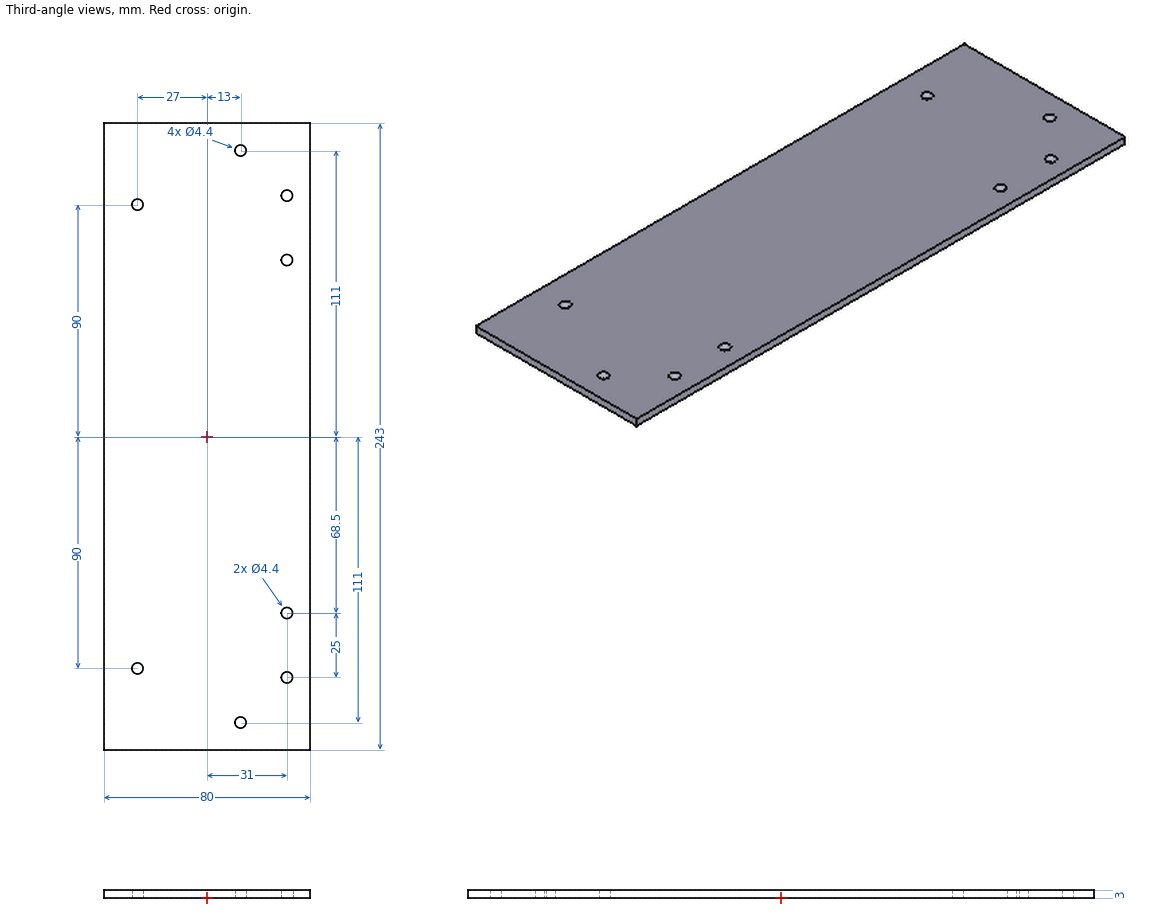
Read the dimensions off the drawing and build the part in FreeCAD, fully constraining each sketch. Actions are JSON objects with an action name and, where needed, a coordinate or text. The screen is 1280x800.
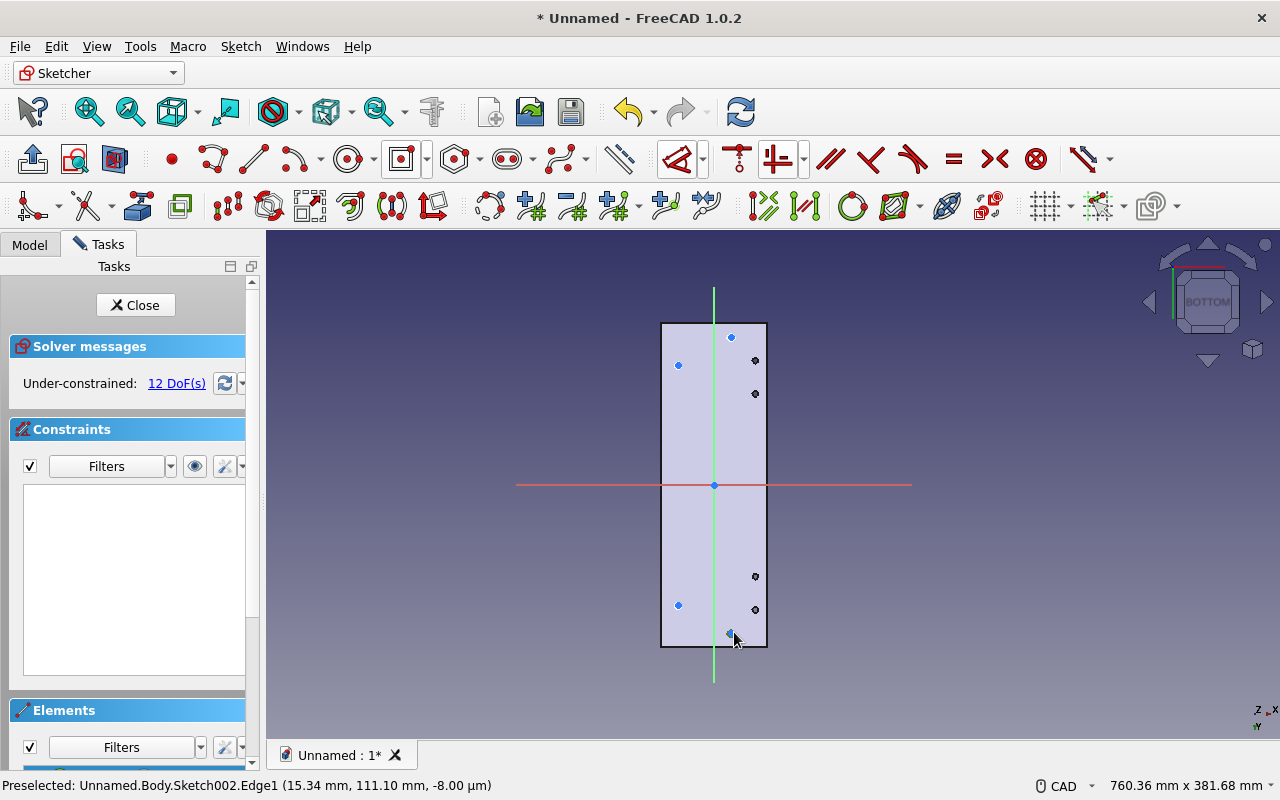
{"action": "scroll", "coordinate": [734, 335], "scroll_direction": "up", "scroll_amount": 7}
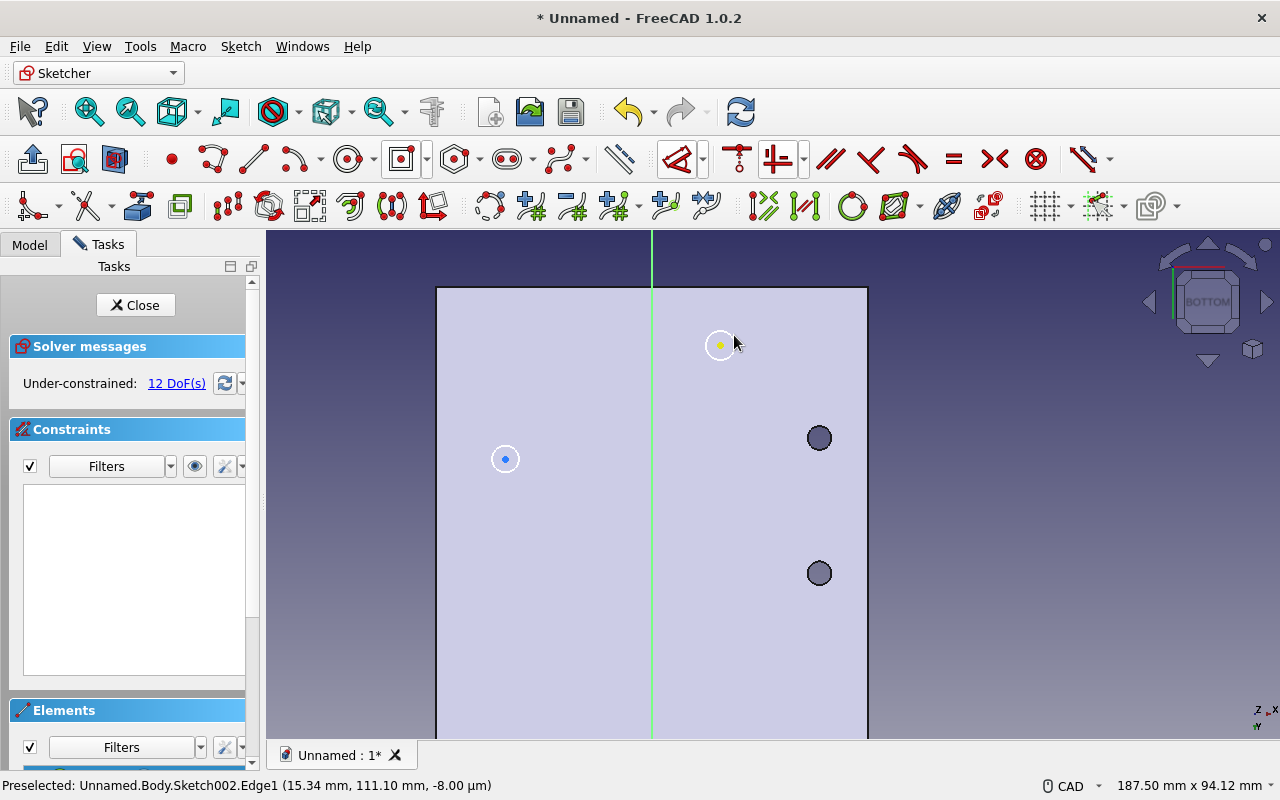
{"action": "left_click", "coordinate": [731, 335]}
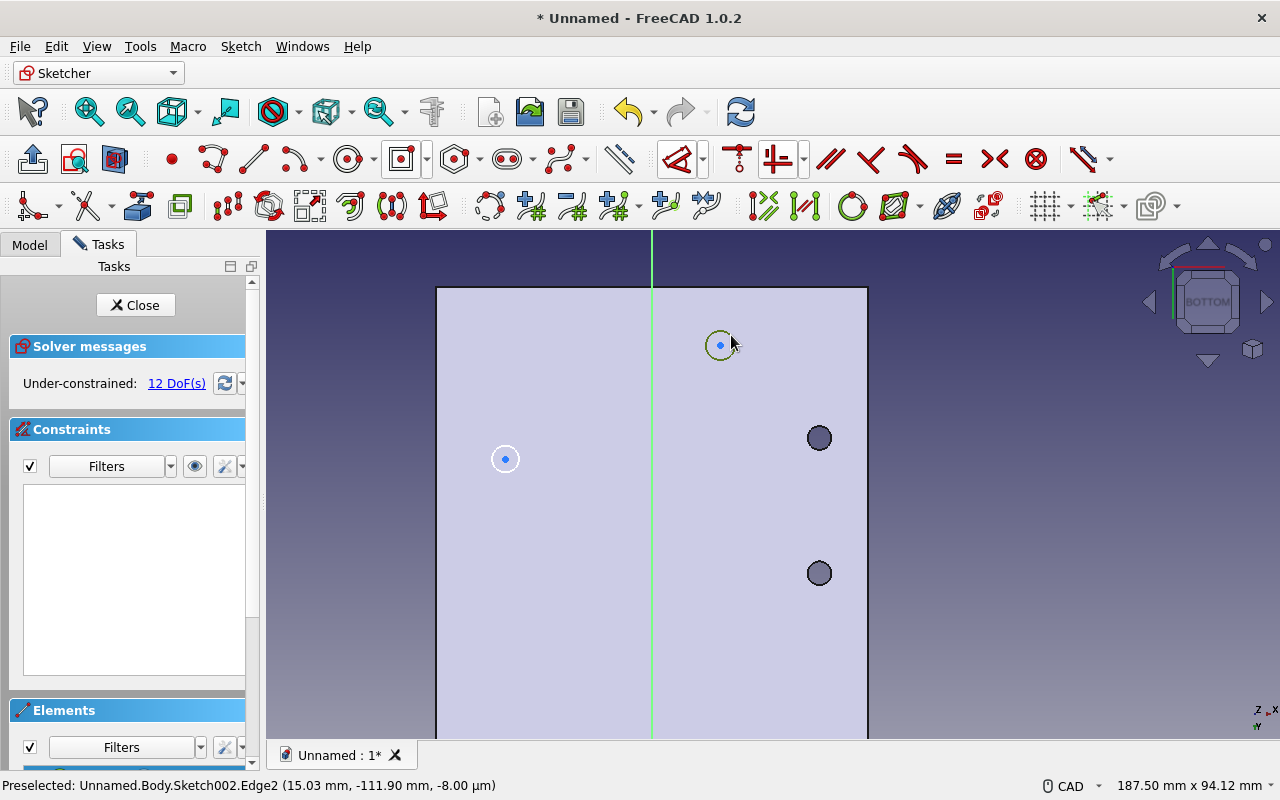
{"action": "scroll", "coordinate": [734, 334], "scroll_direction": "down", "scroll_amount": 7}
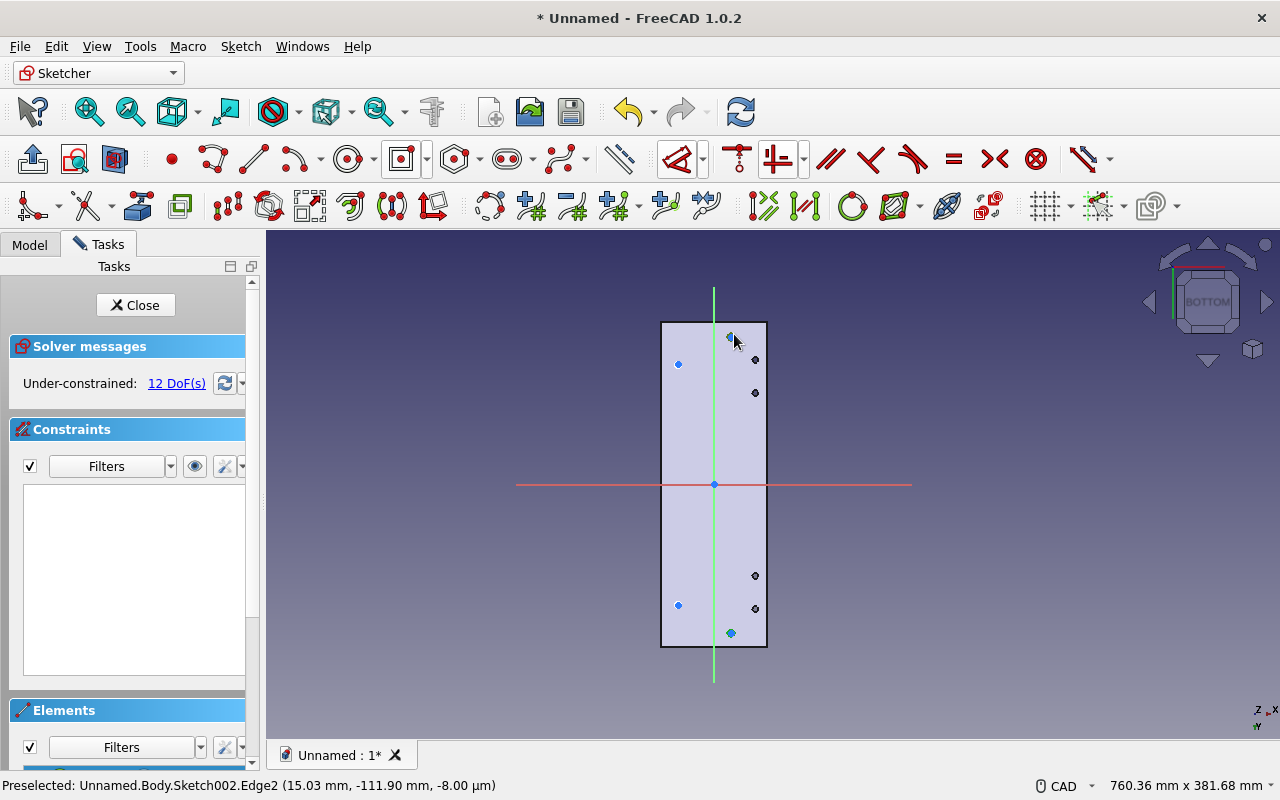
{"action": "scroll", "coordinate": [680, 603], "scroll_direction": "up", "scroll_amount": 8}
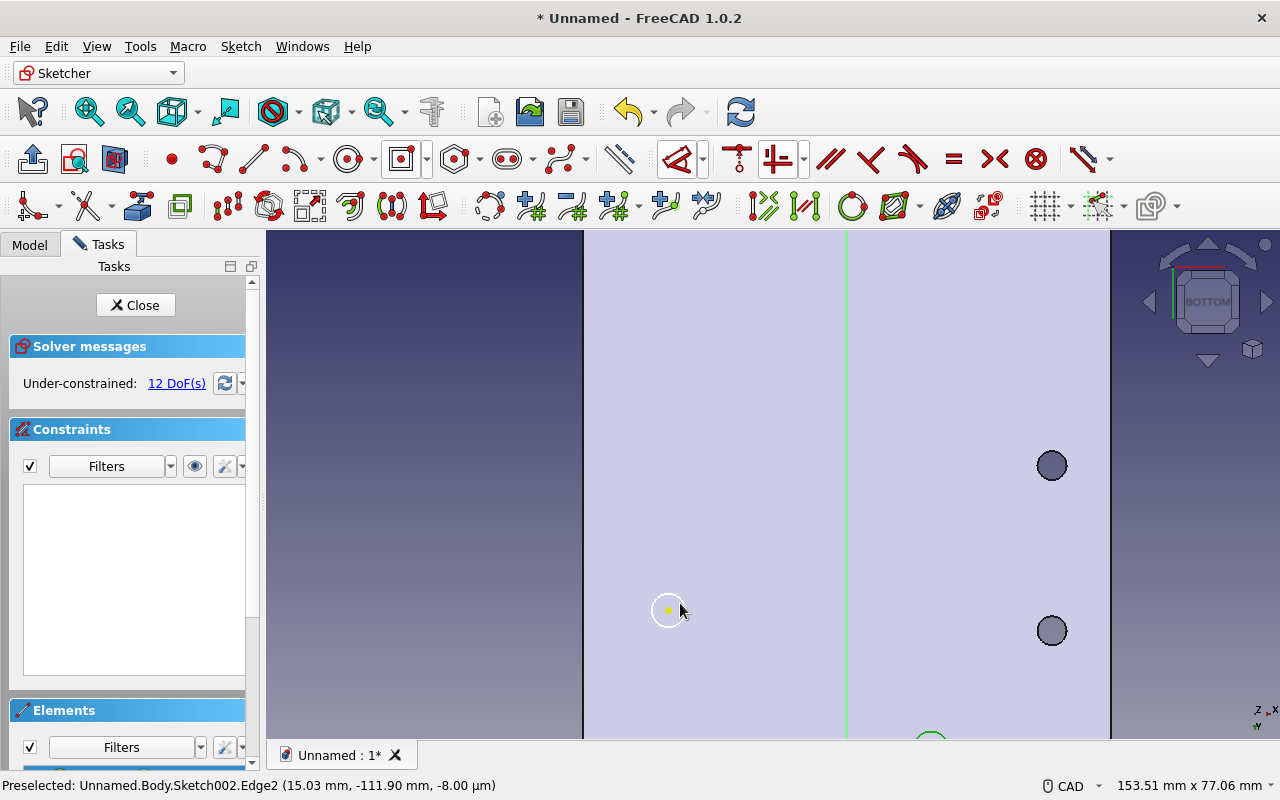
{"action": "left_click", "coordinate": [680, 599]}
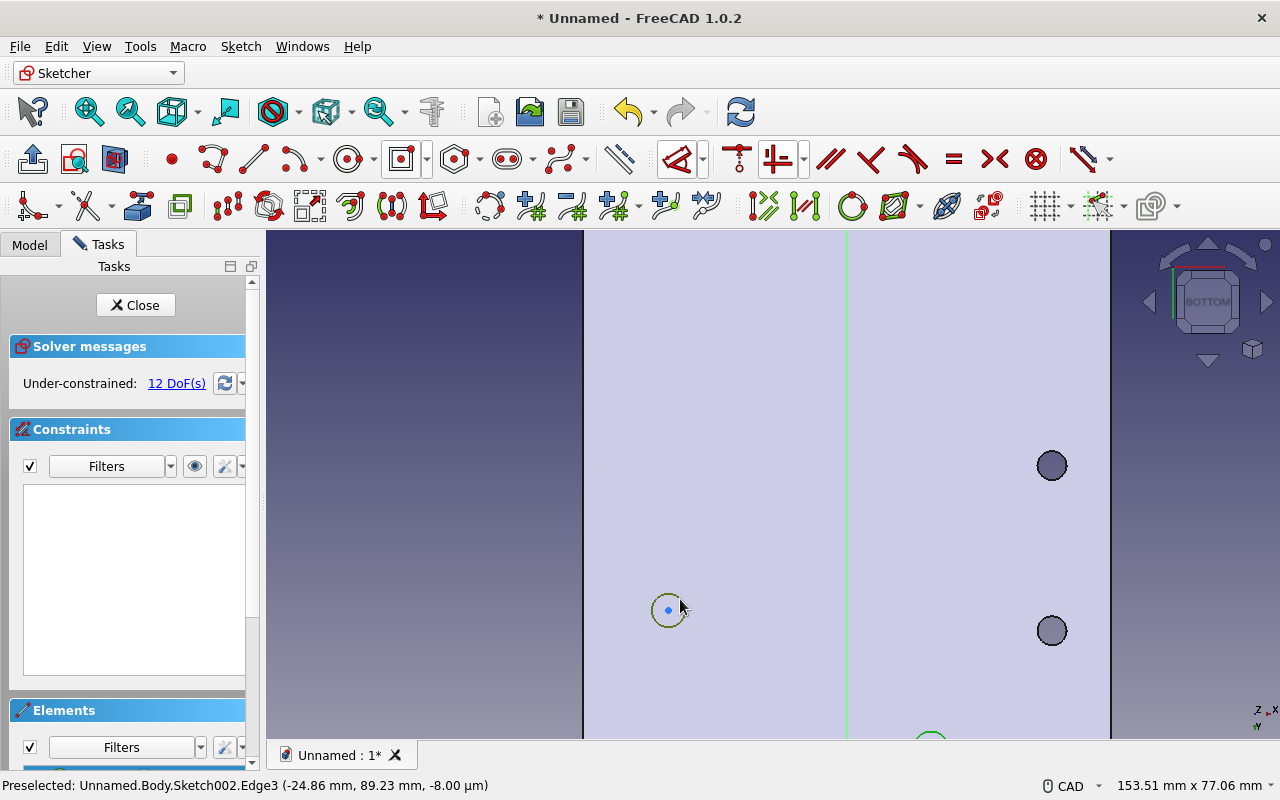
{"action": "scroll", "coordinate": [680, 604], "scroll_direction": "down", "scroll_amount": 8}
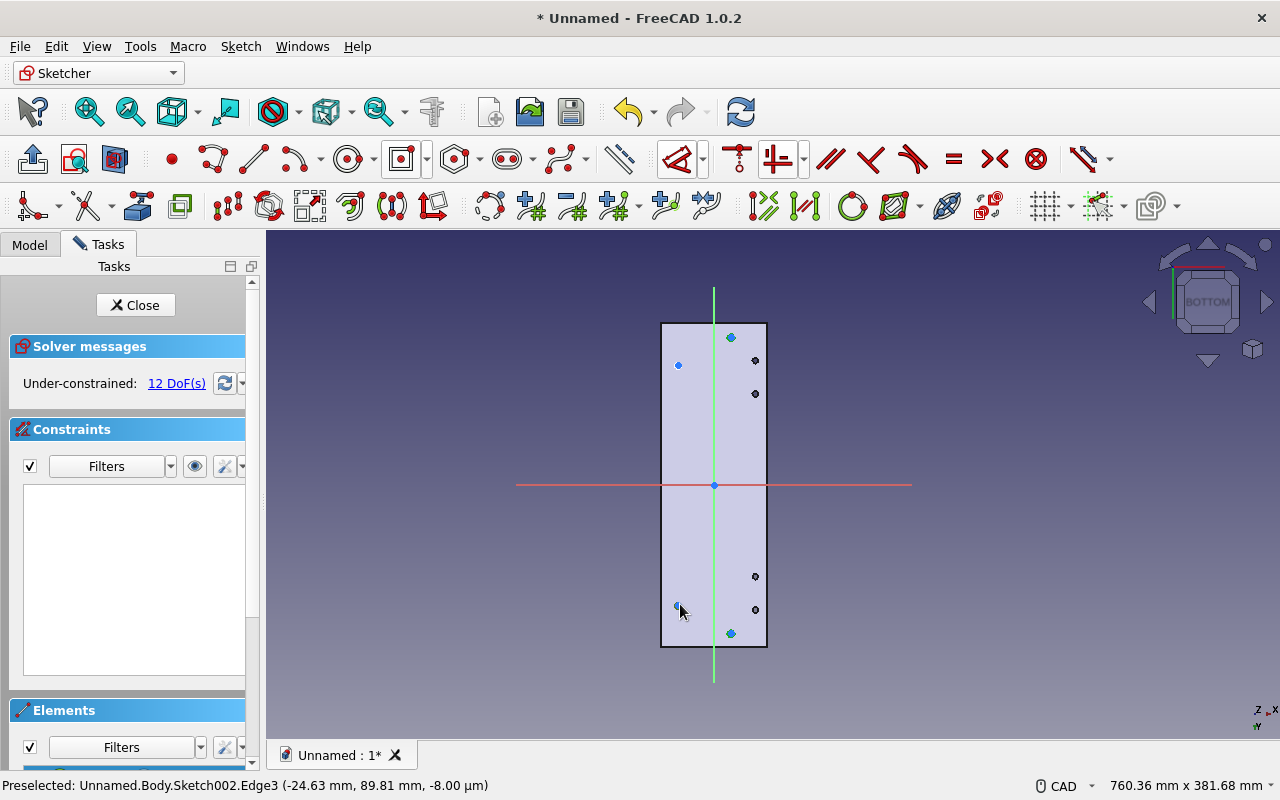
{"action": "scroll", "coordinate": [680, 363], "scroll_direction": "up", "scroll_amount": 8}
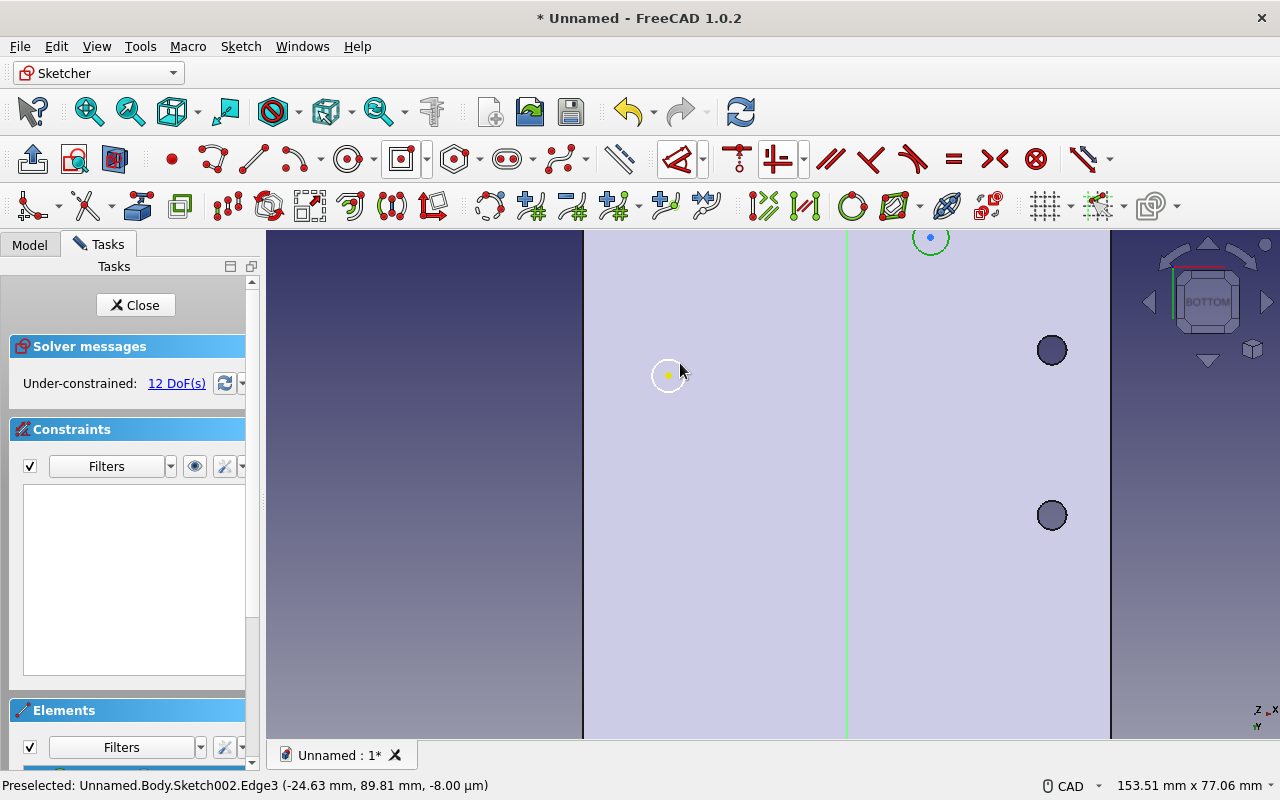
{"action": "left_click", "coordinate": [680, 364]}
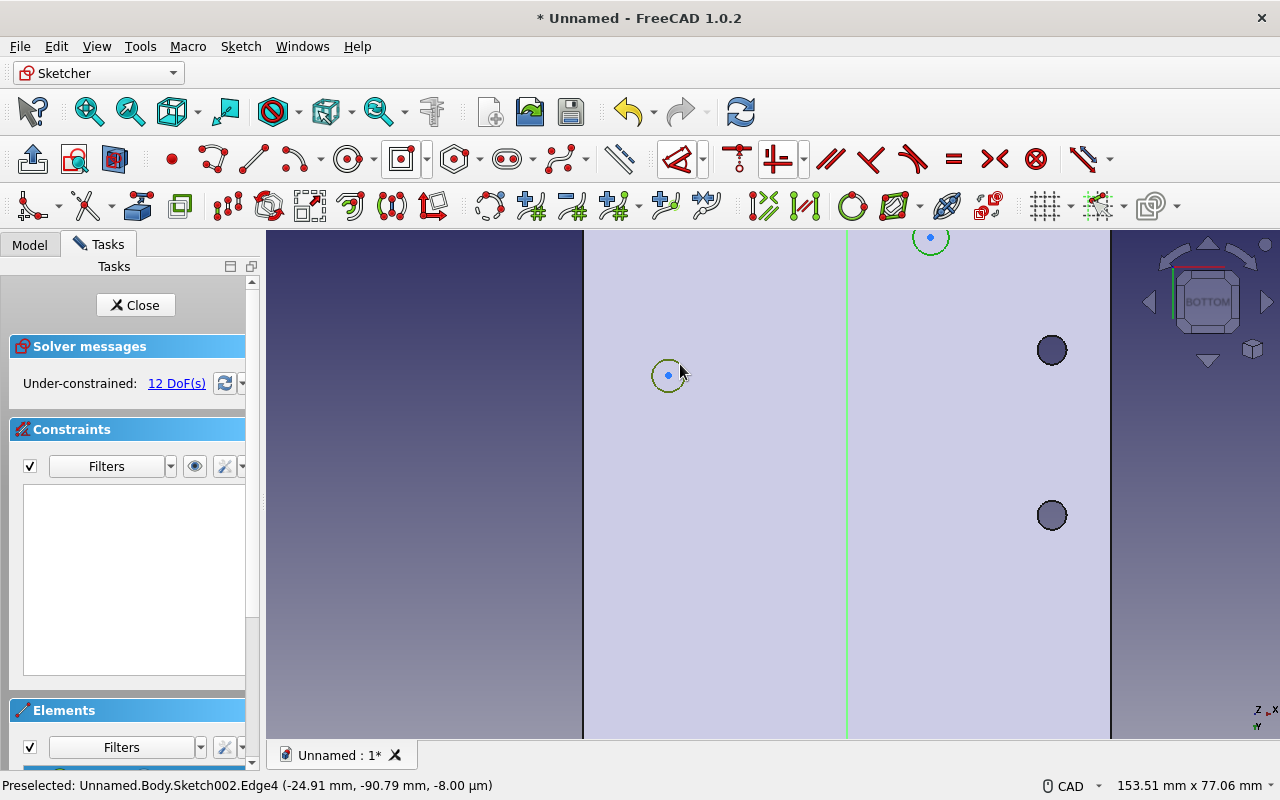
{"action": "left_click", "coordinate": [954, 160]}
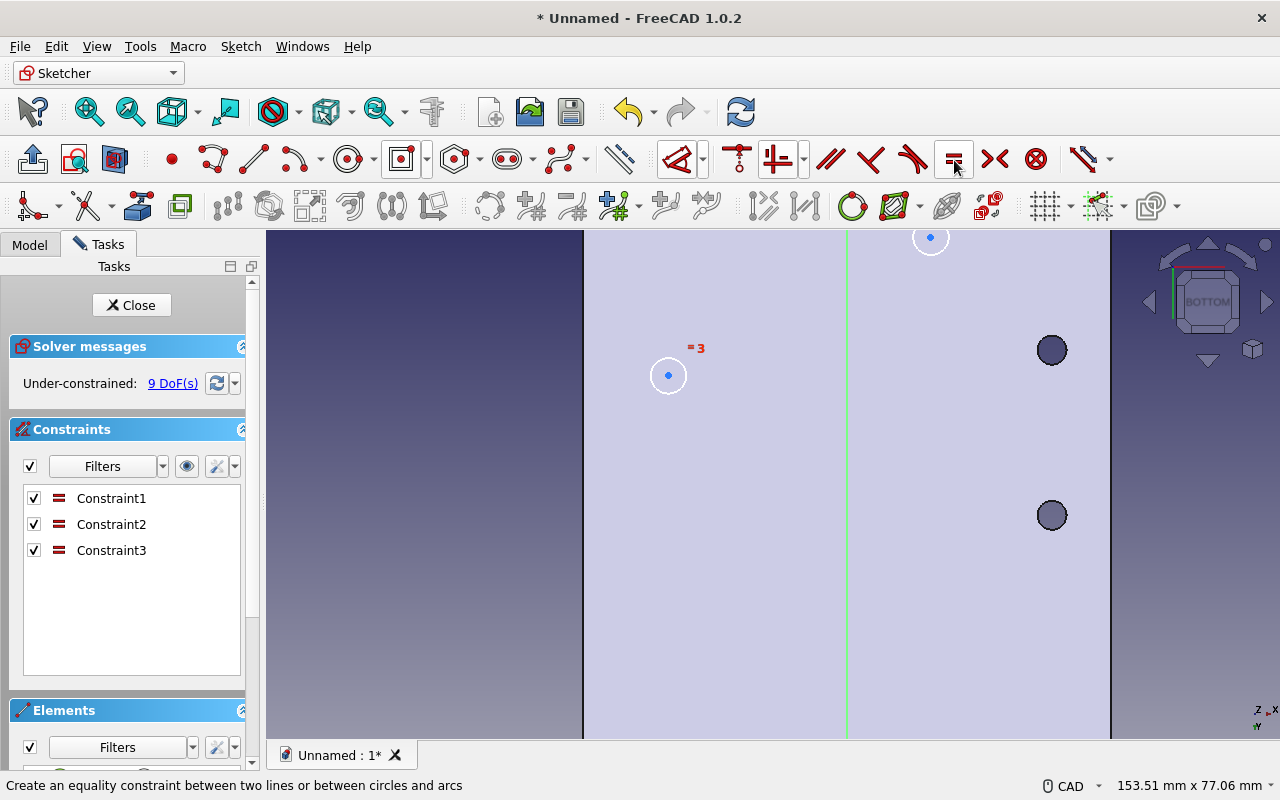
{"action": "scroll", "coordinate": [680, 362], "scroll_direction": "down", "scroll_amount": 8}